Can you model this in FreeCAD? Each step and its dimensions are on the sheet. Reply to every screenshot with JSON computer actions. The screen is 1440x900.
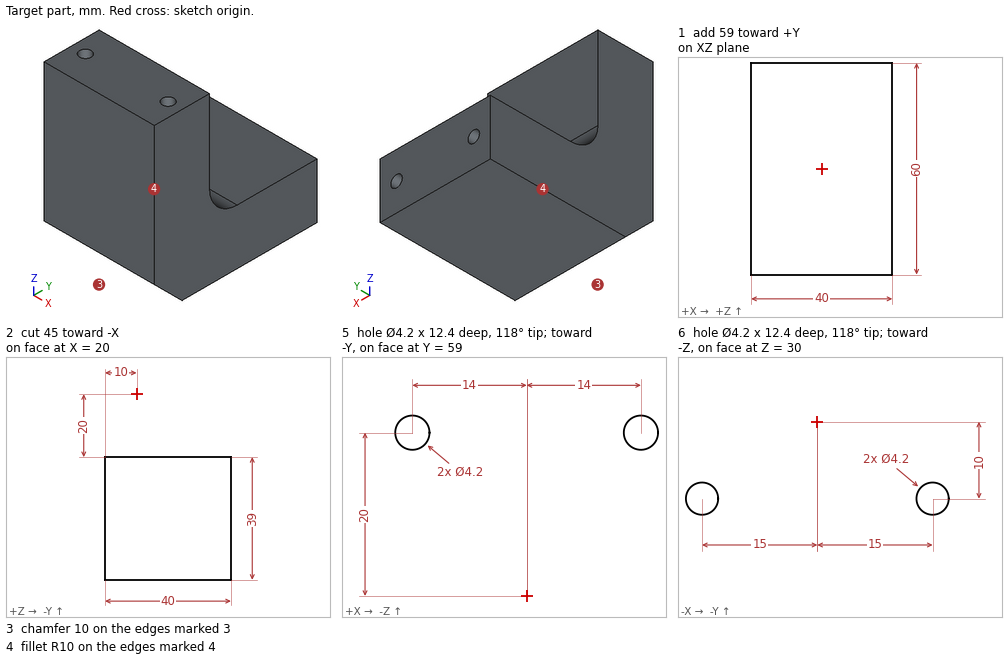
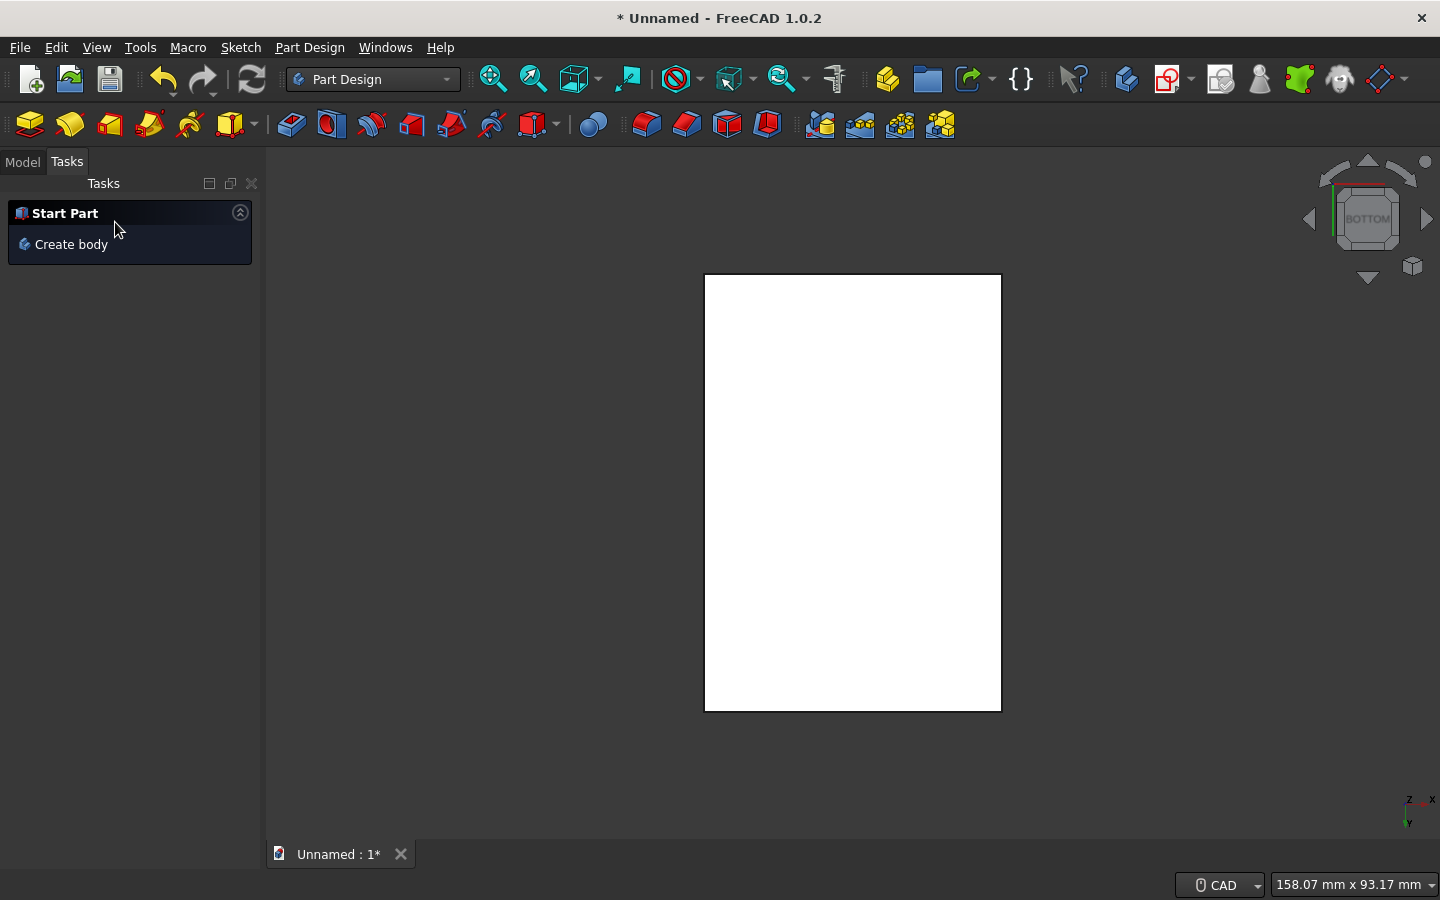
{"action": "left_click", "coordinate": [853, 273]}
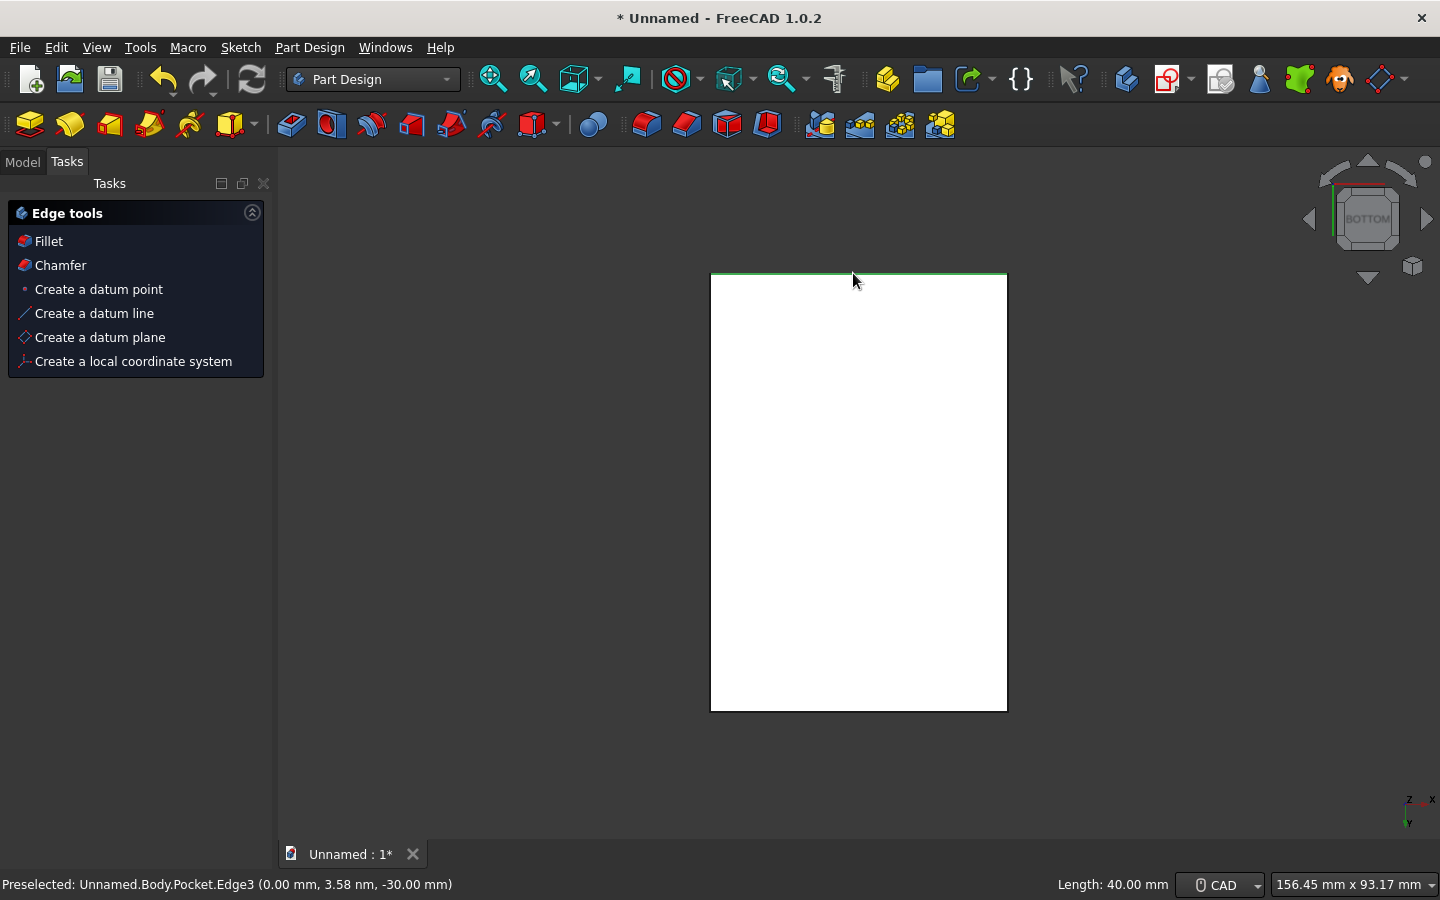
{"action": "left_click", "coordinate": [688, 124]}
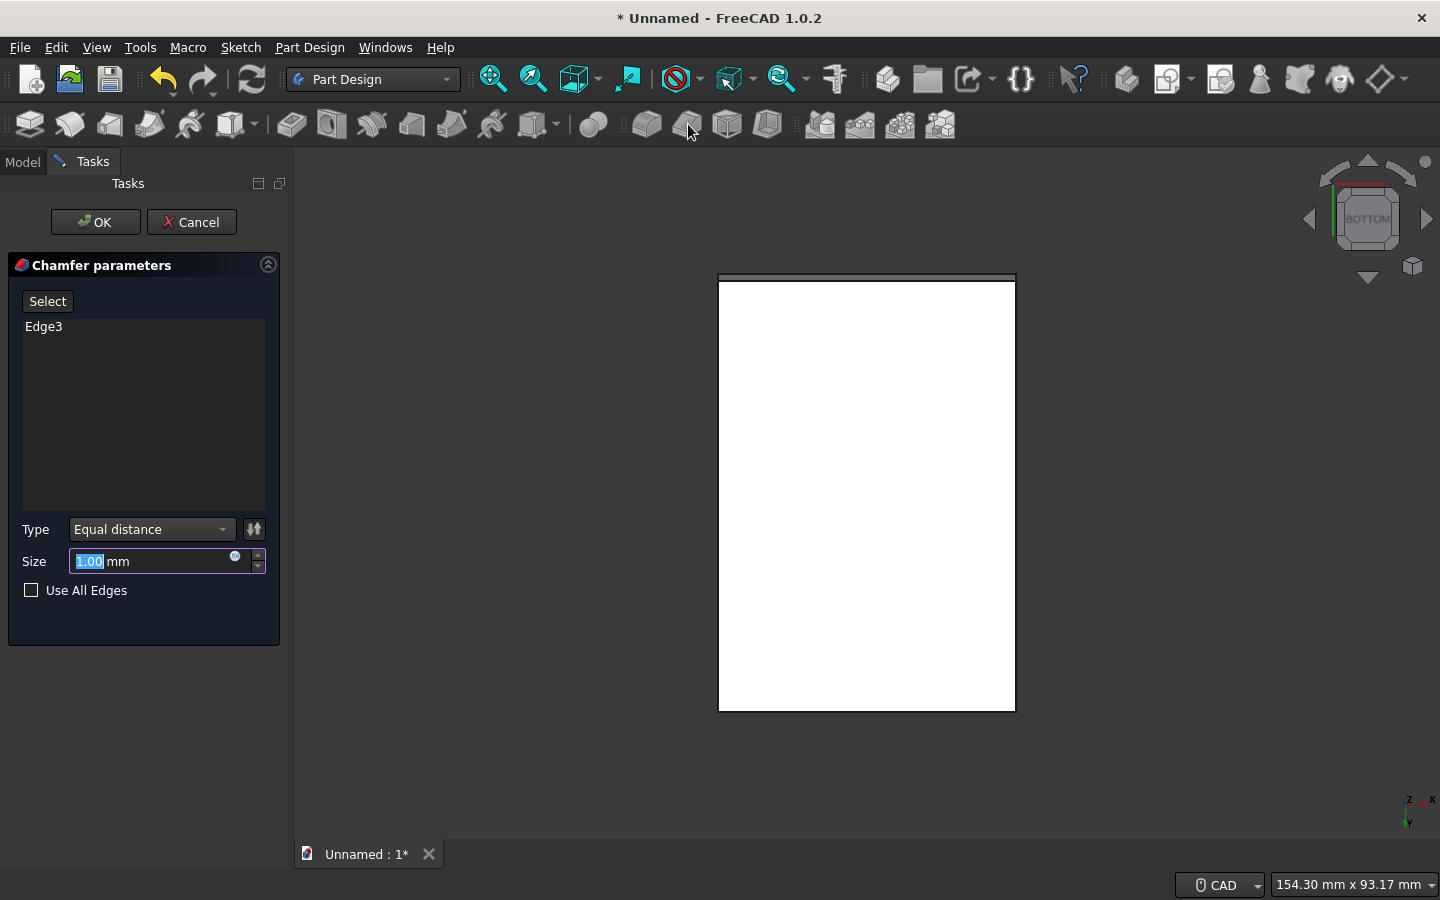
{"action": "type", "text": "10"}
{"action": "key", "text": "Tab"}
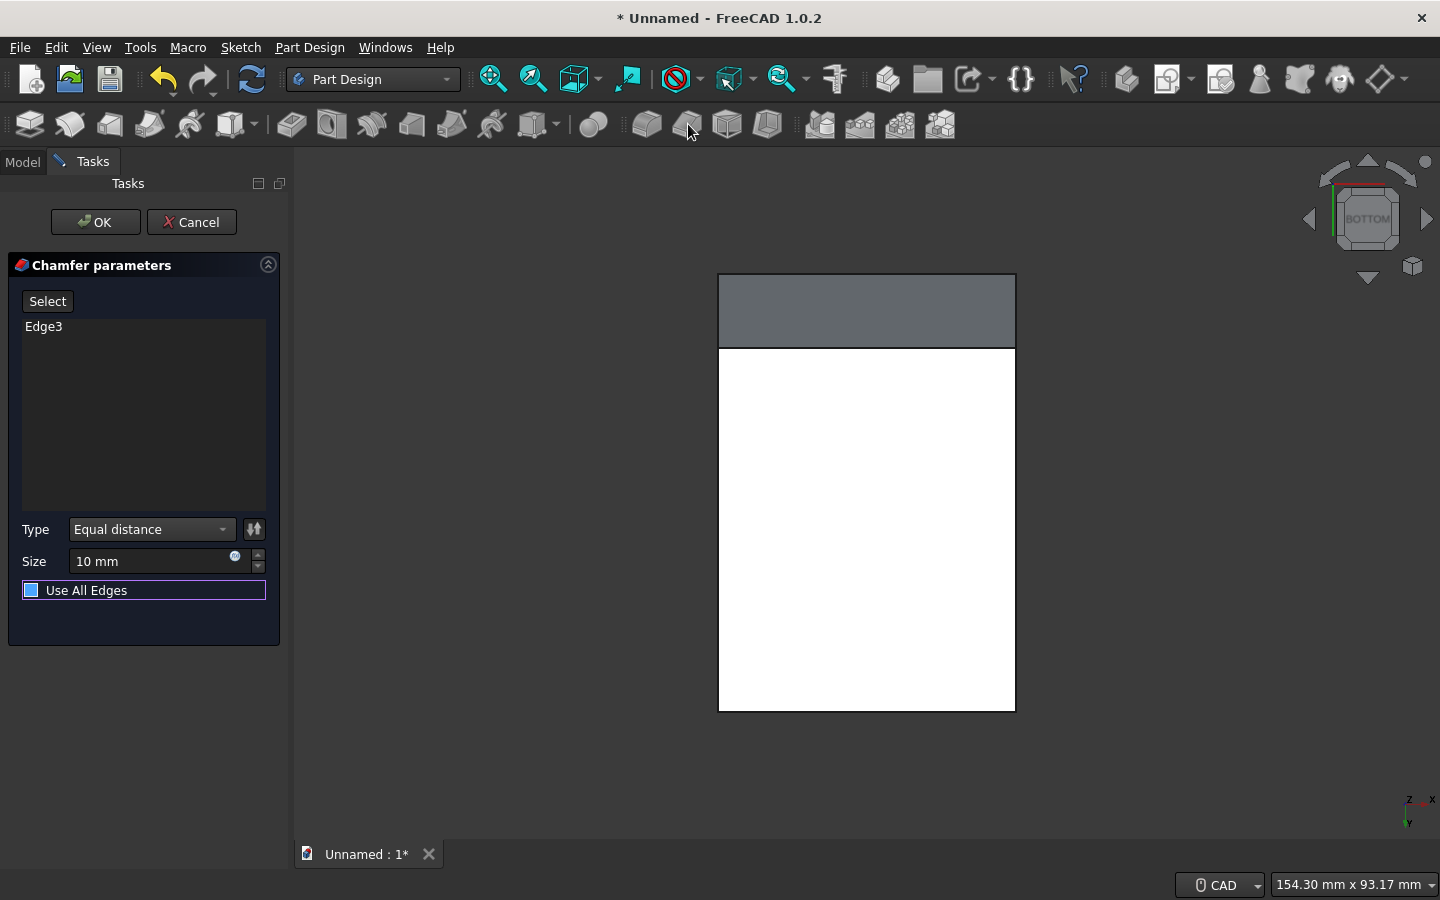
{"action": "left_click", "coordinate": [96, 222]}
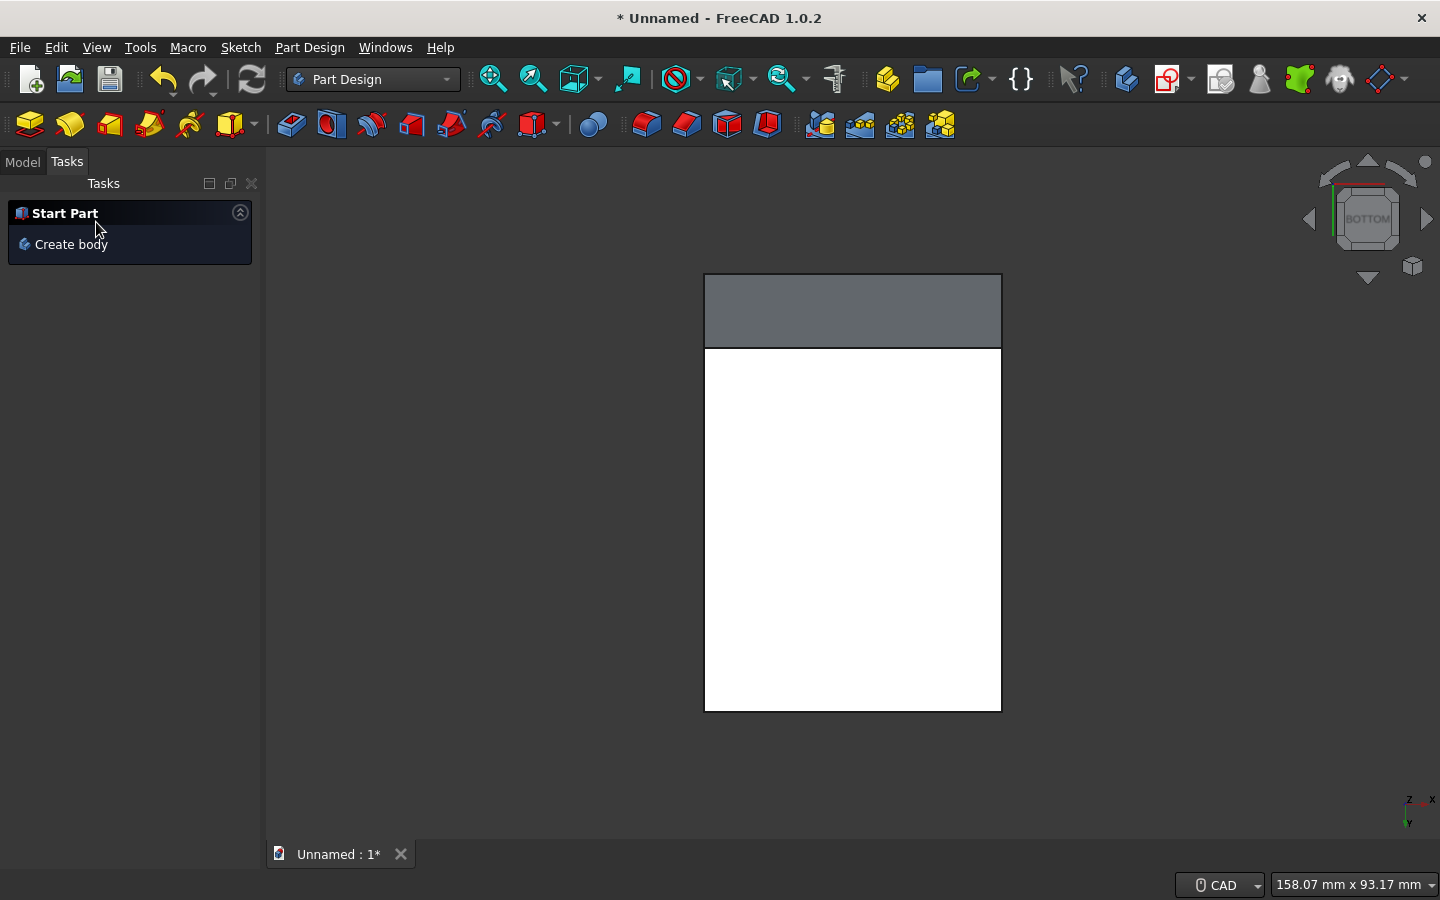
{"action": "key", "text": "0"}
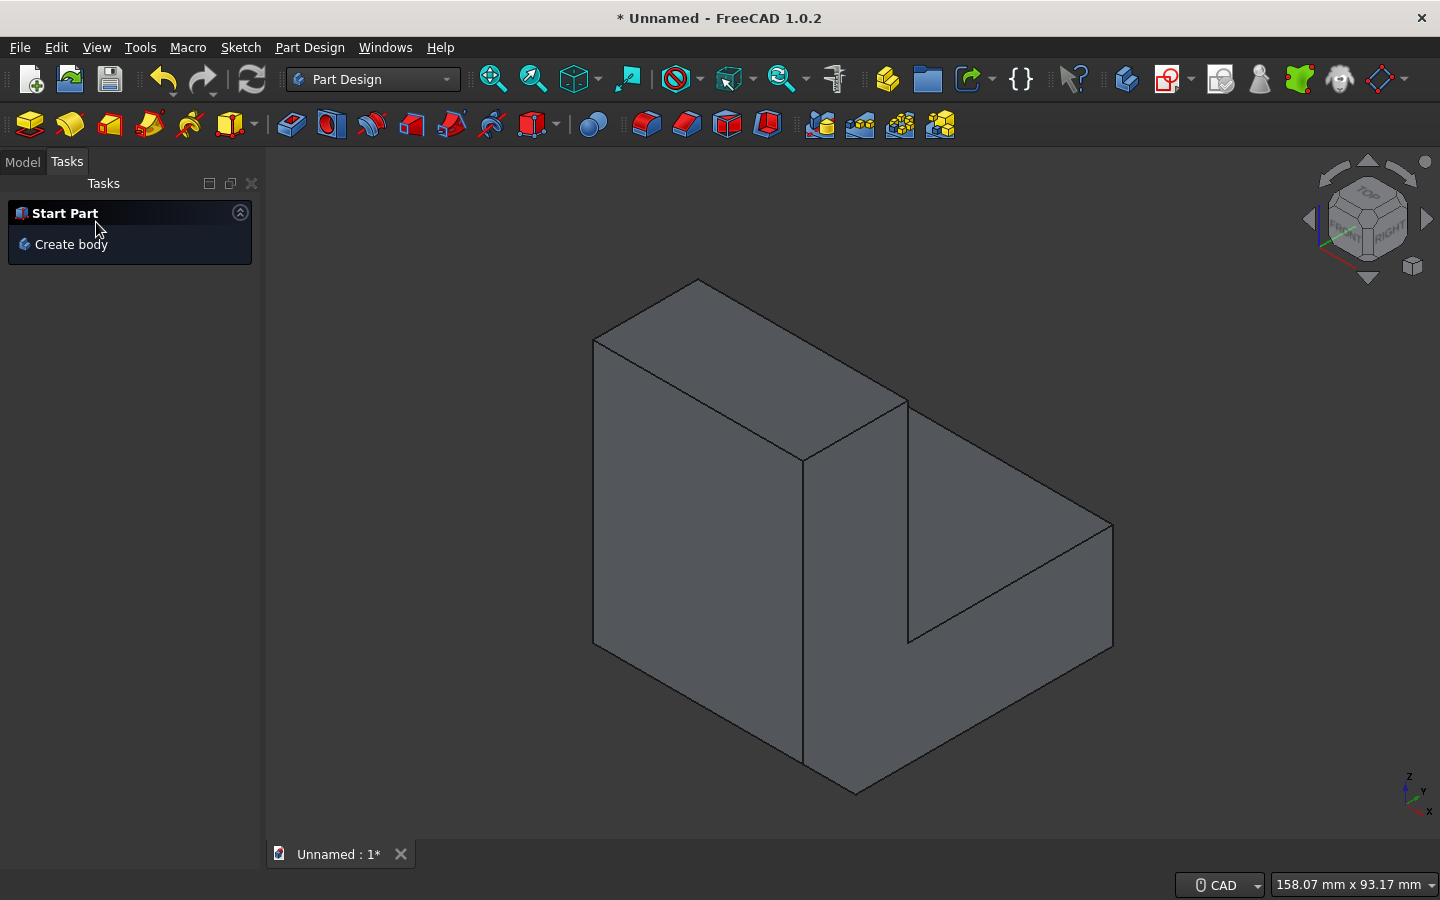
{"action": "key", "text": "2"}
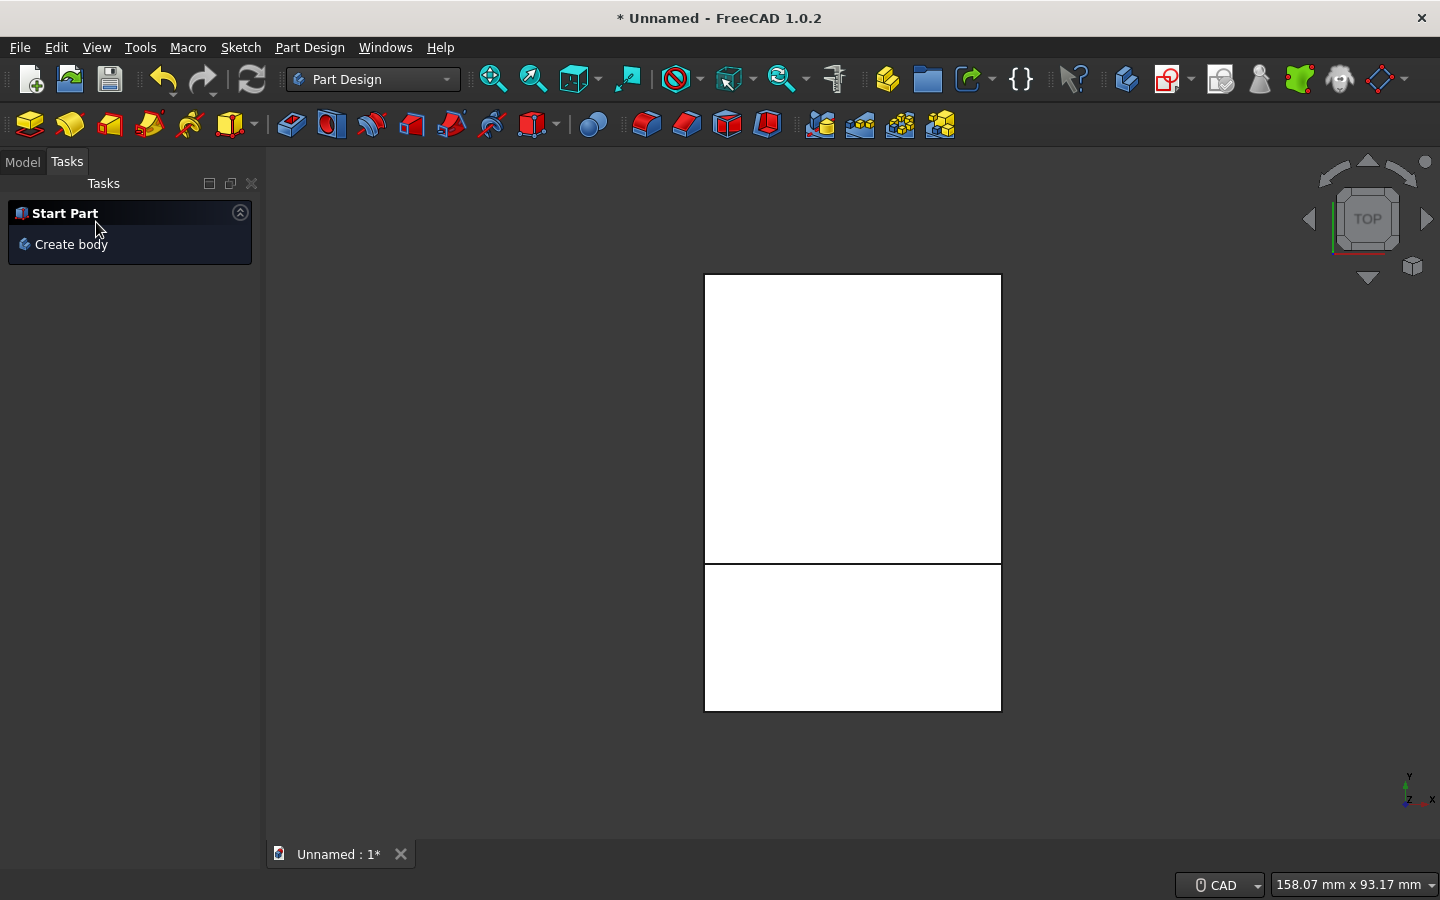
{"action": "key", "text": "1"}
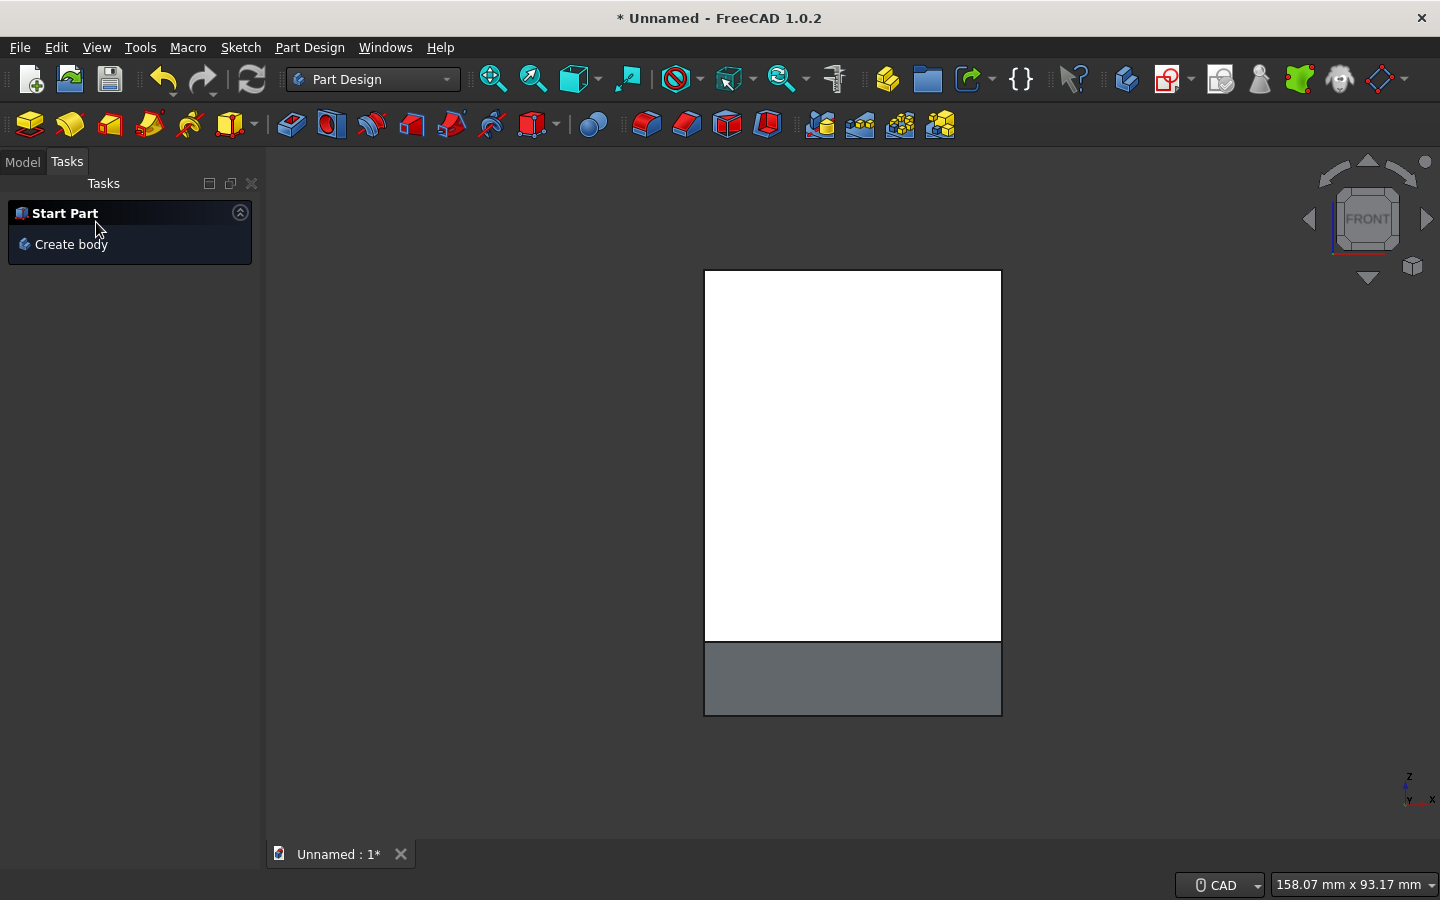
{"action": "key", "text": "3"}